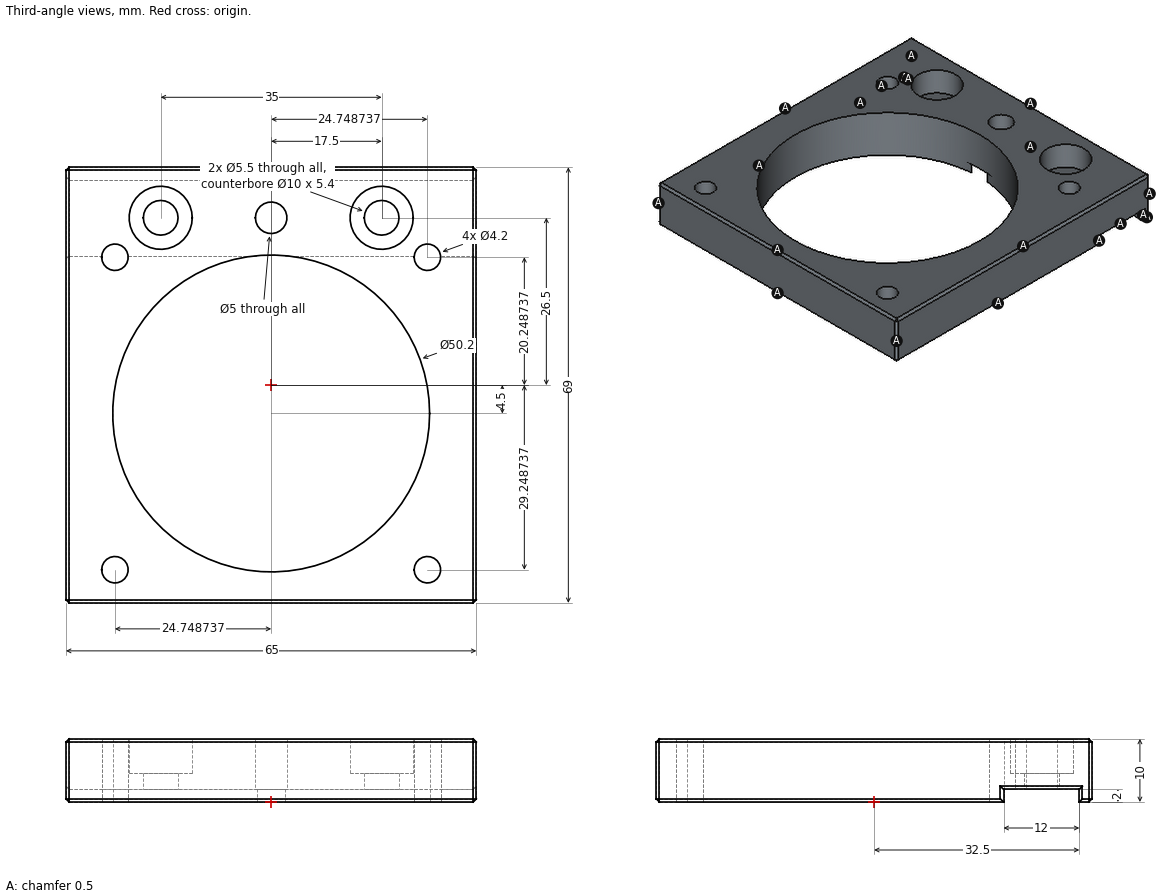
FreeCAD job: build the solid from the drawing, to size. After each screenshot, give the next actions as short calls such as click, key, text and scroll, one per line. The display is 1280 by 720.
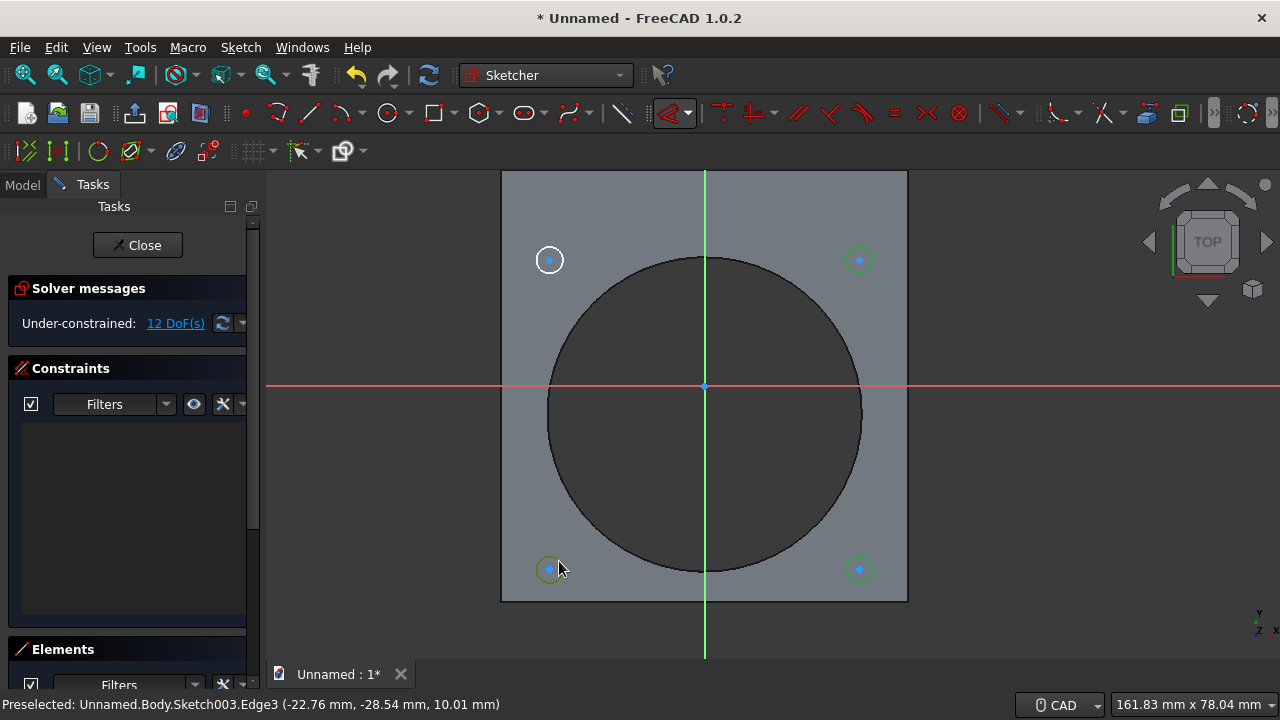
click(559, 251)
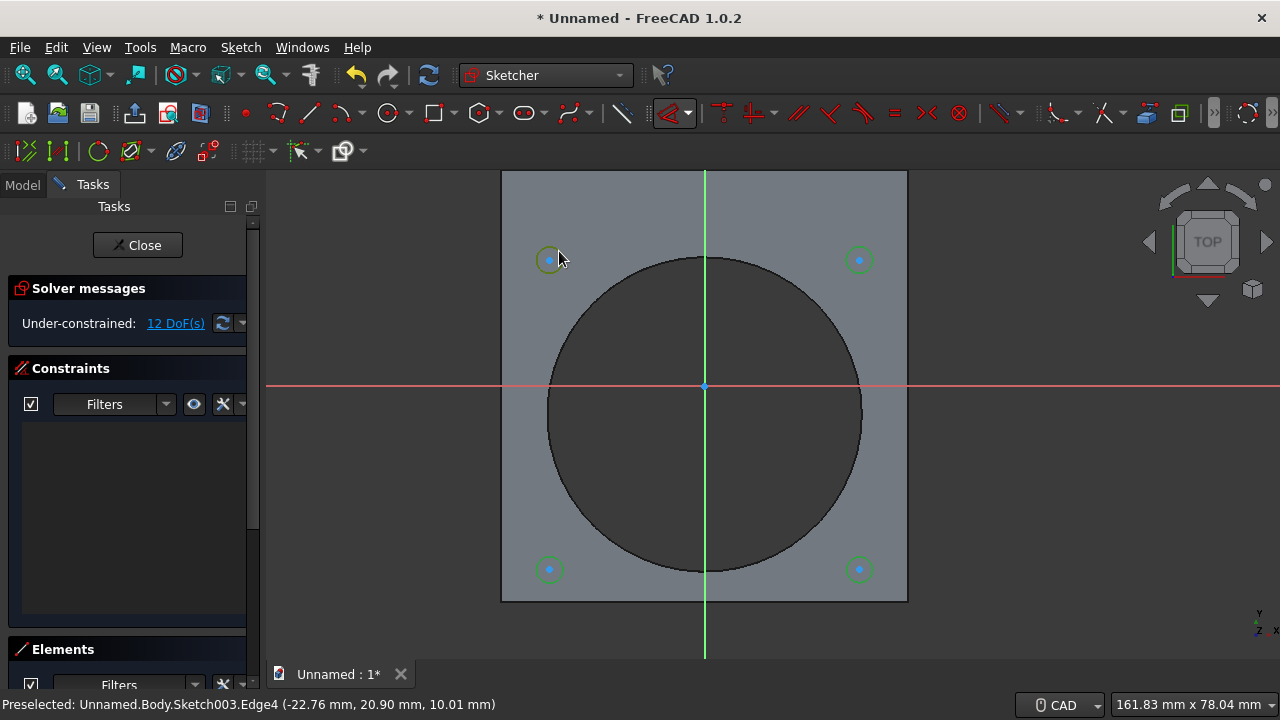
click(896, 114)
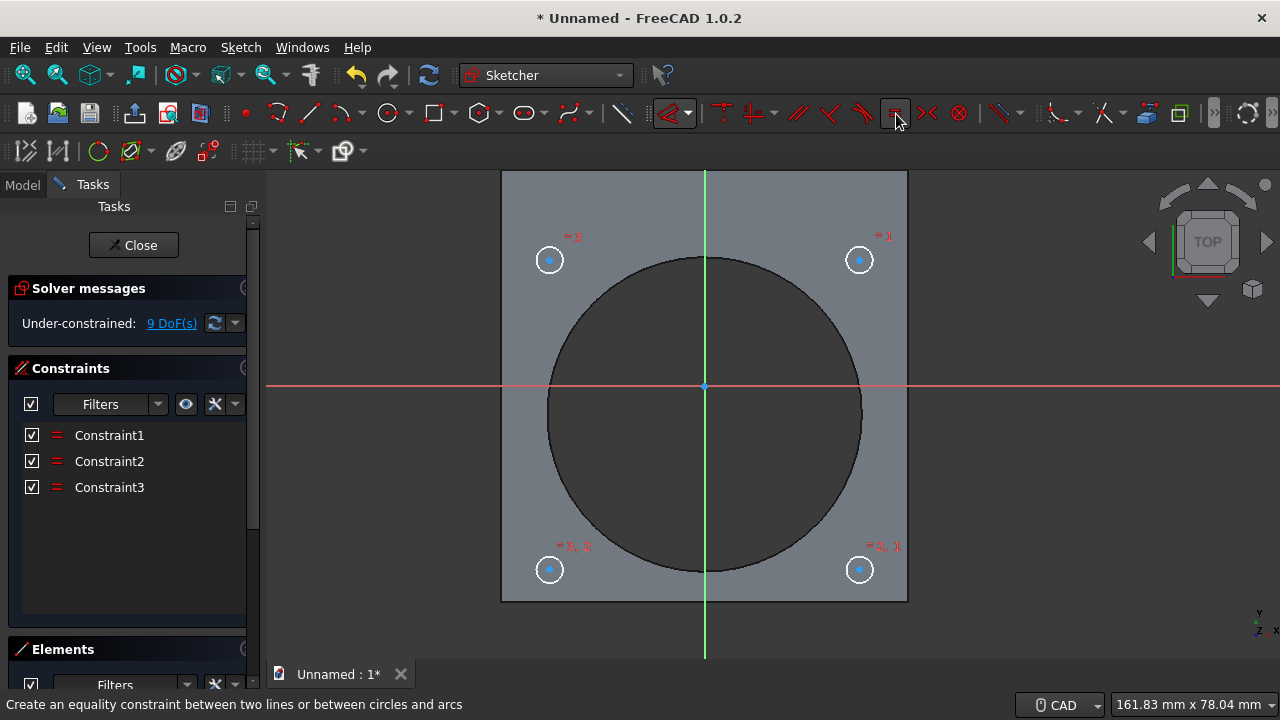
click(860, 260)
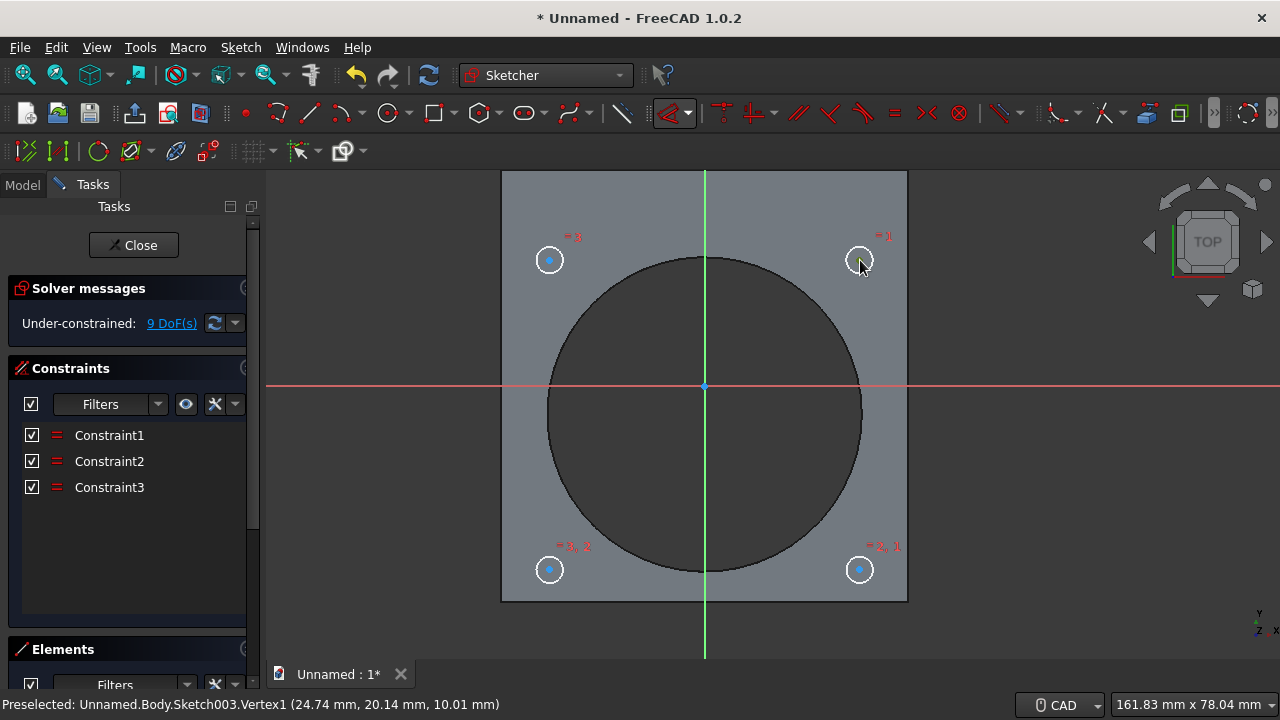
click(860, 570)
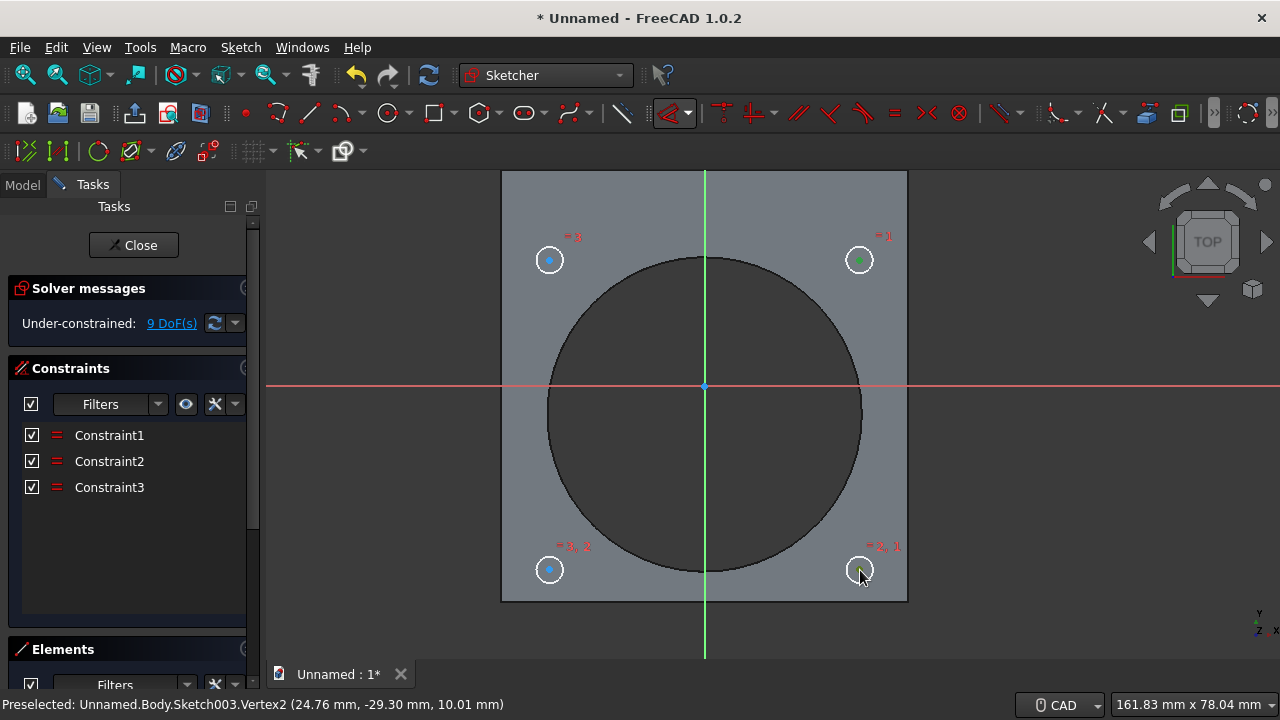
key(v)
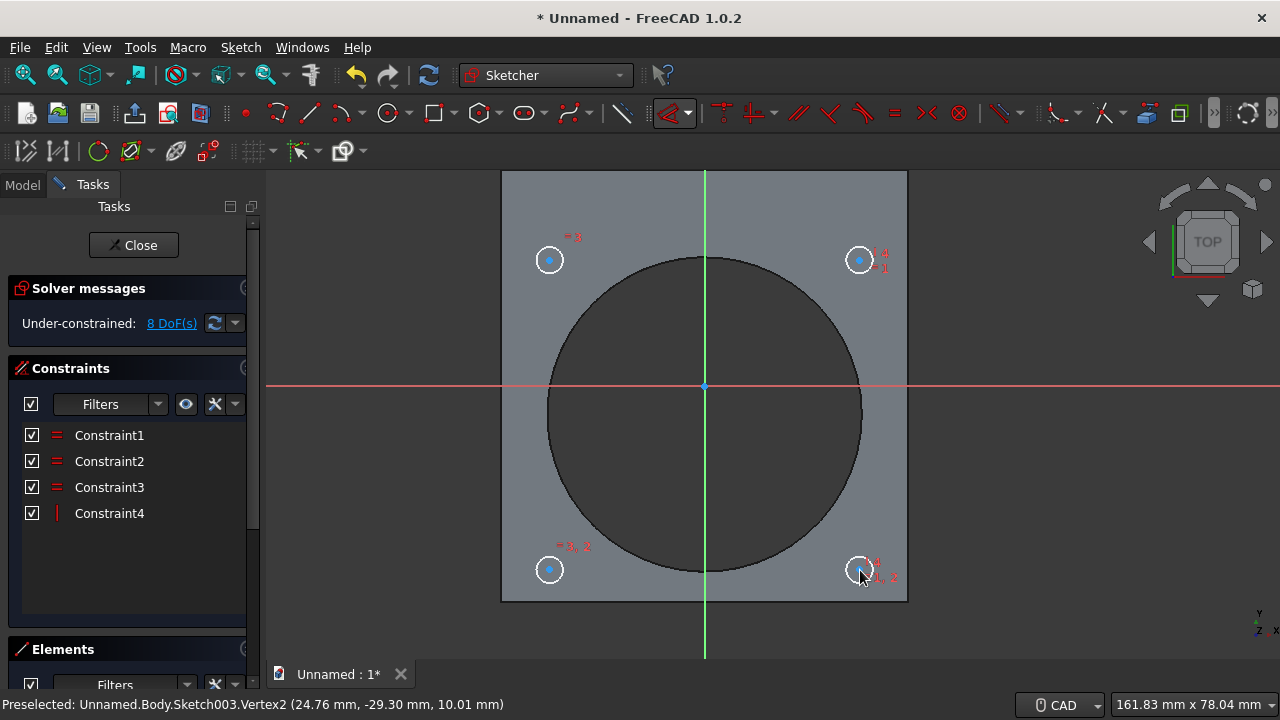
click(860, 570)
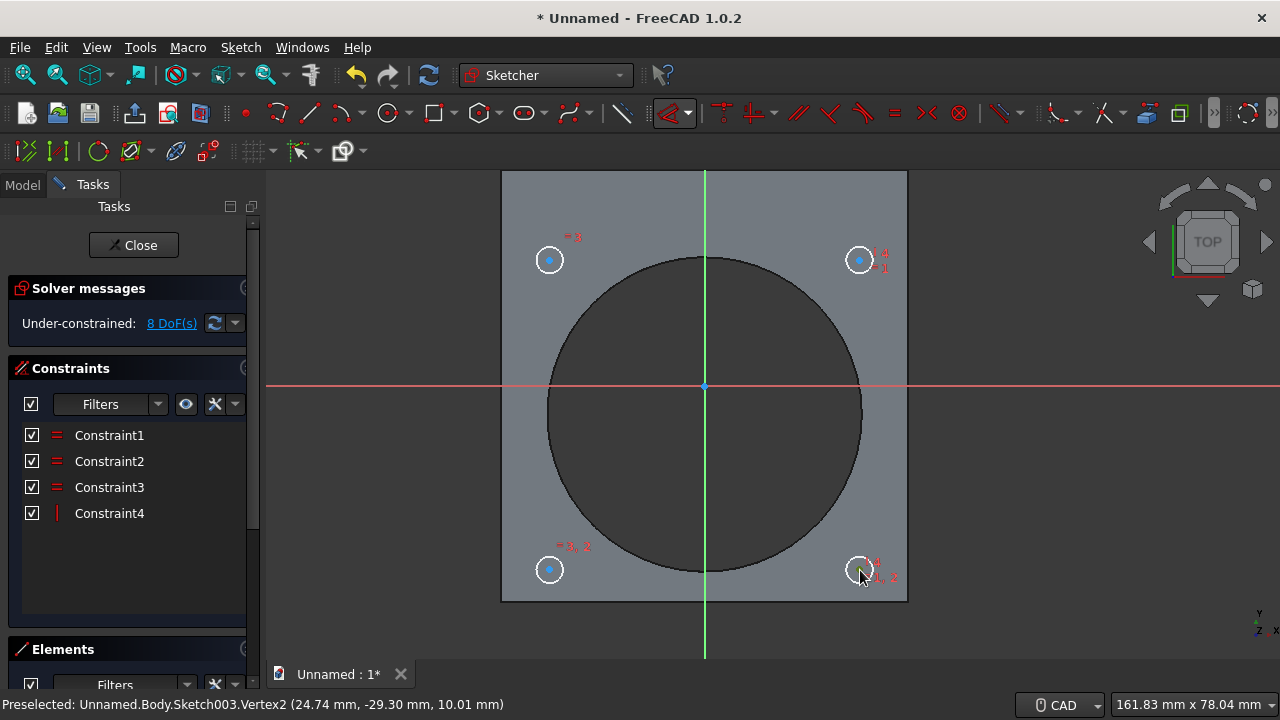
click(550, 570)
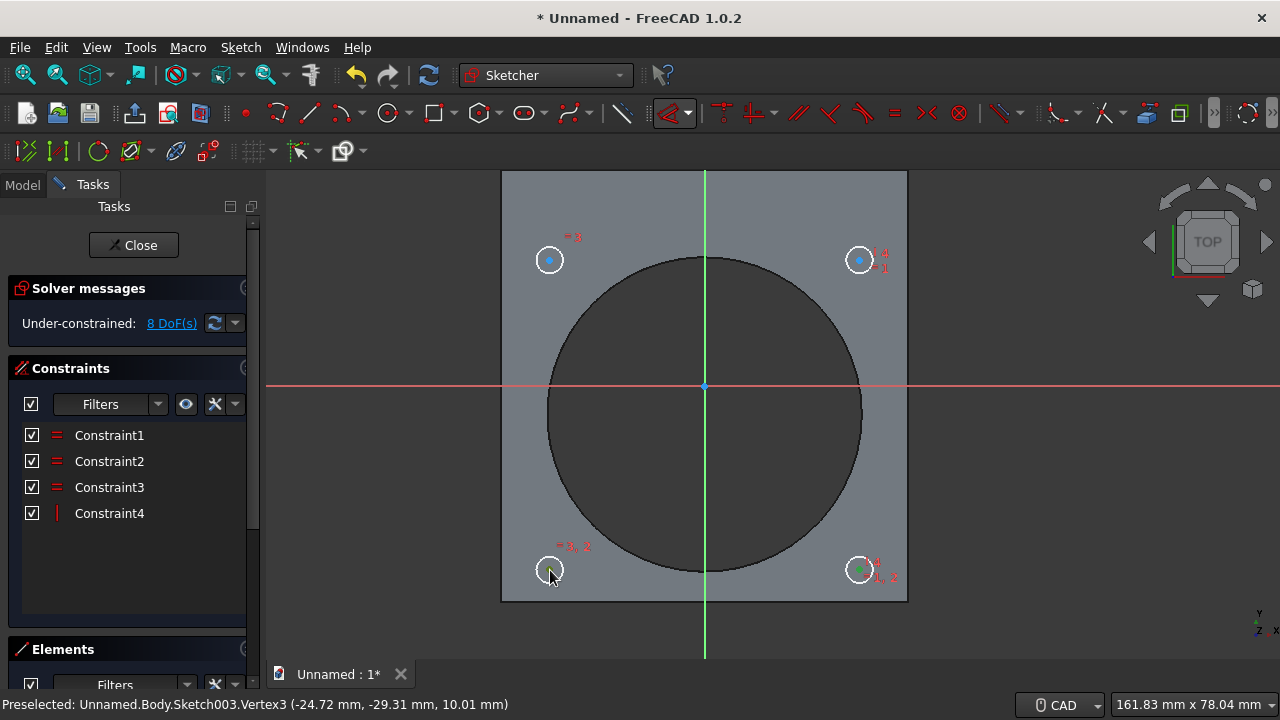
key(h)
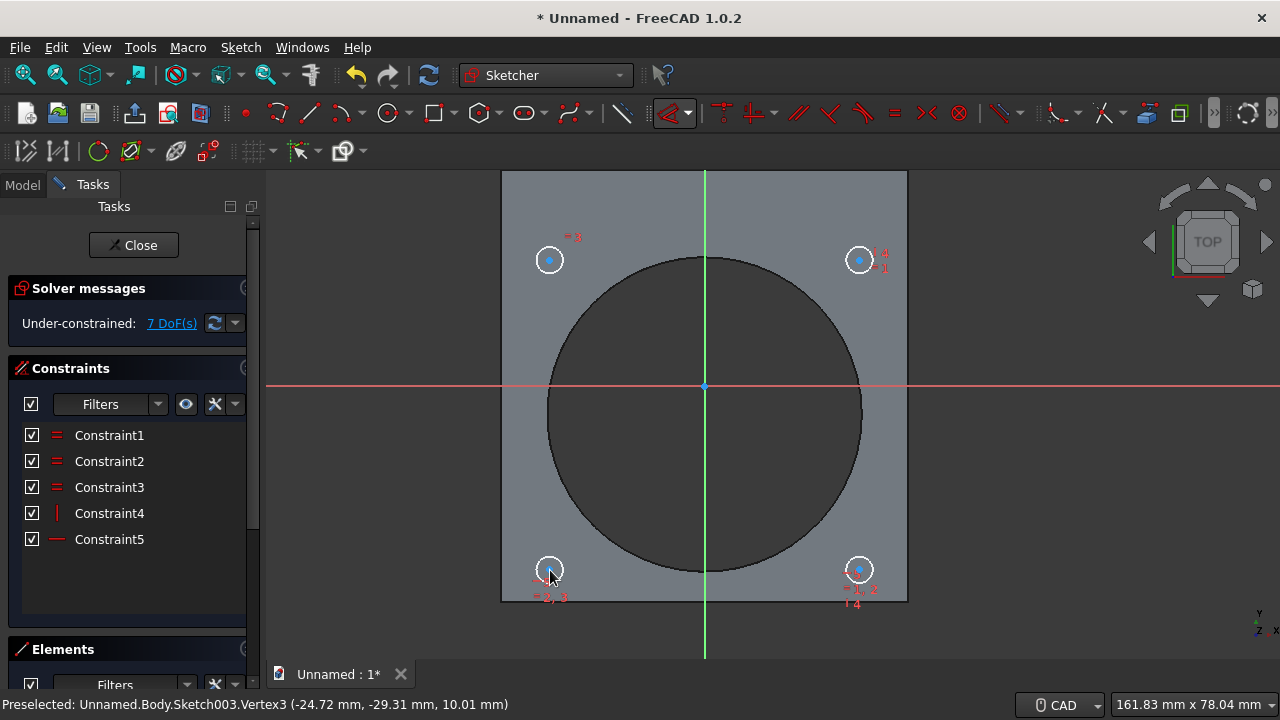
click(550, 570)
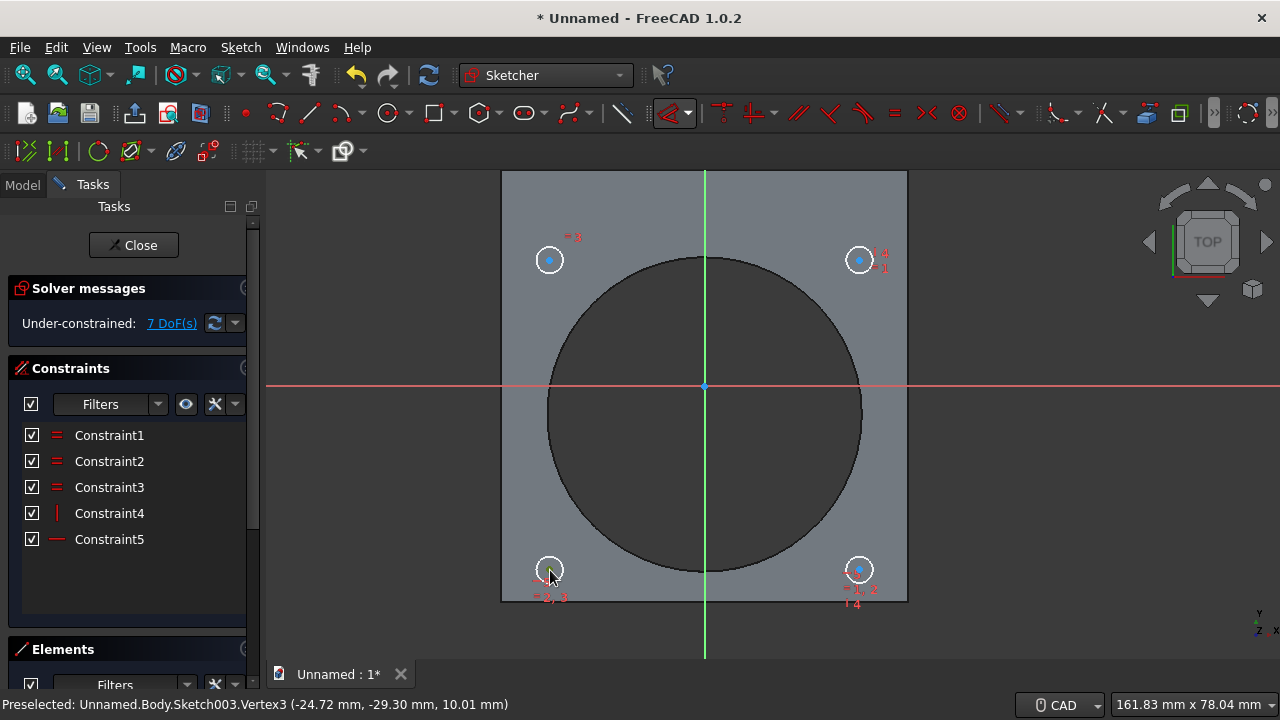
click(550, 260)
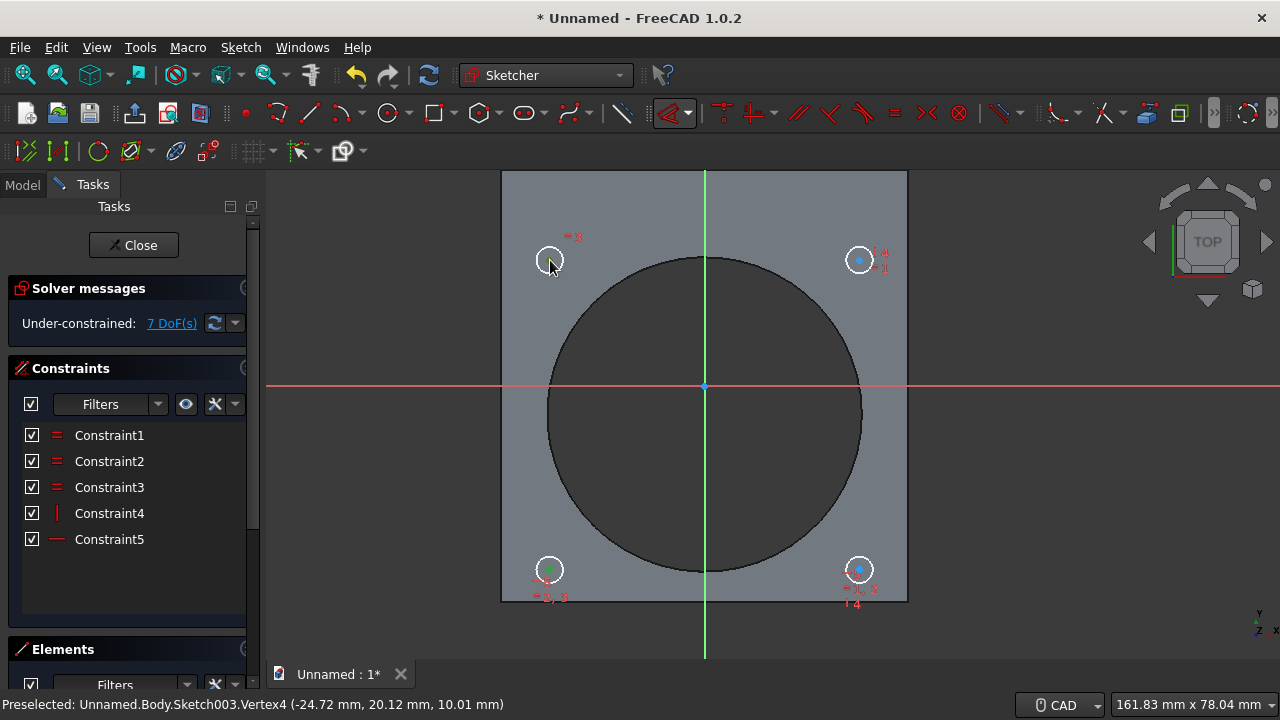
key(v)